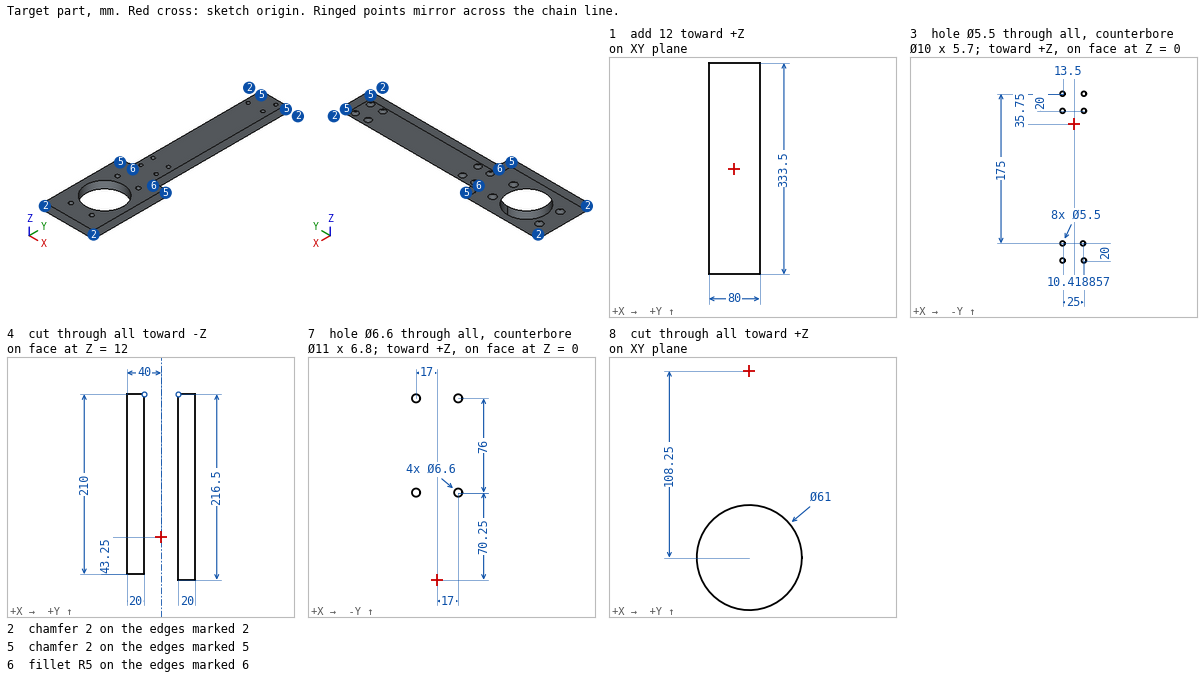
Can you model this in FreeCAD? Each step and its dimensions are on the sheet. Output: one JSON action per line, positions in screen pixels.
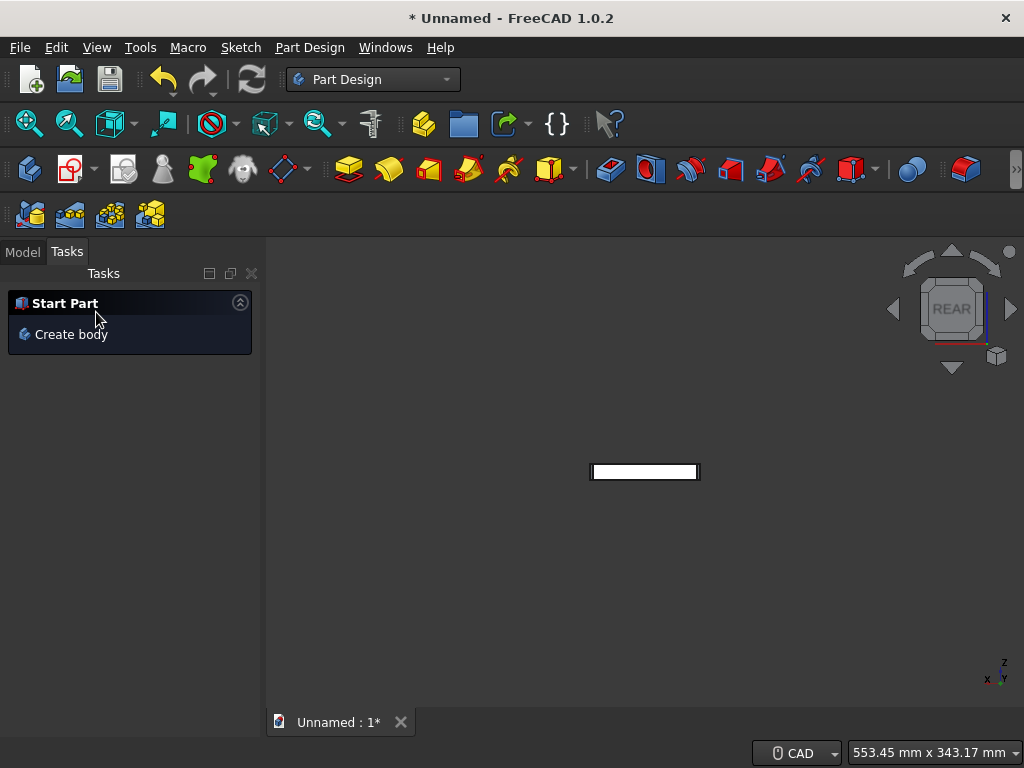
{"action": "key", "text": "5"}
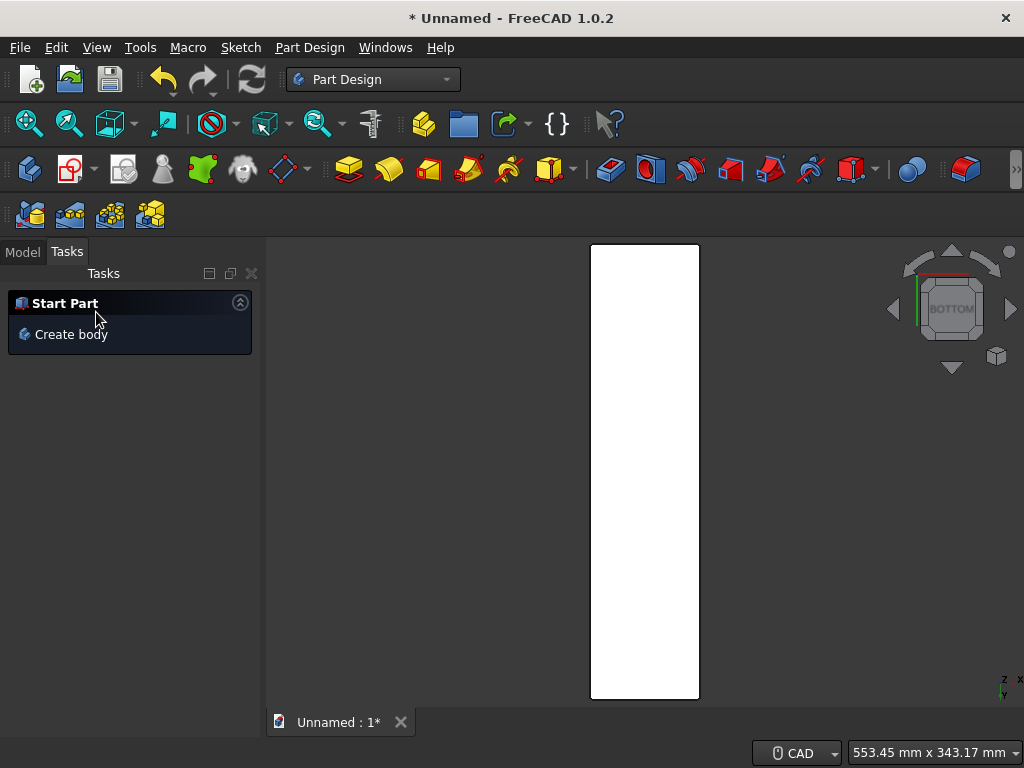
{"action": "left_click", "coordinate": [645, 602]}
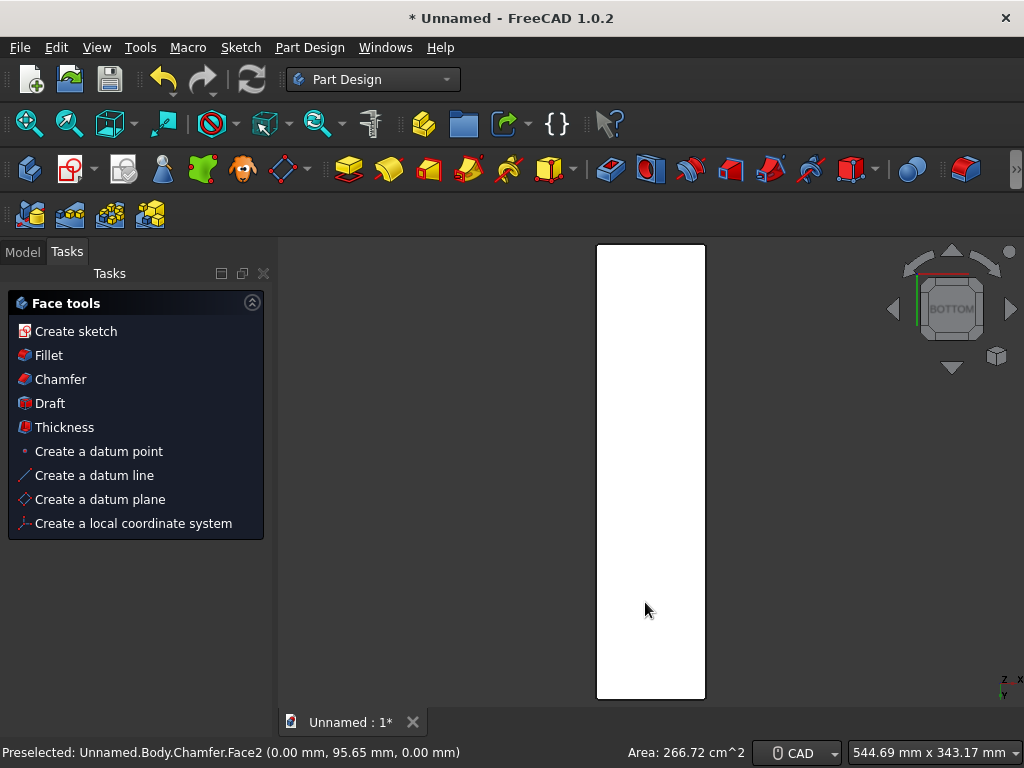
{"action": "left_click", "coordinate": [70, 170]}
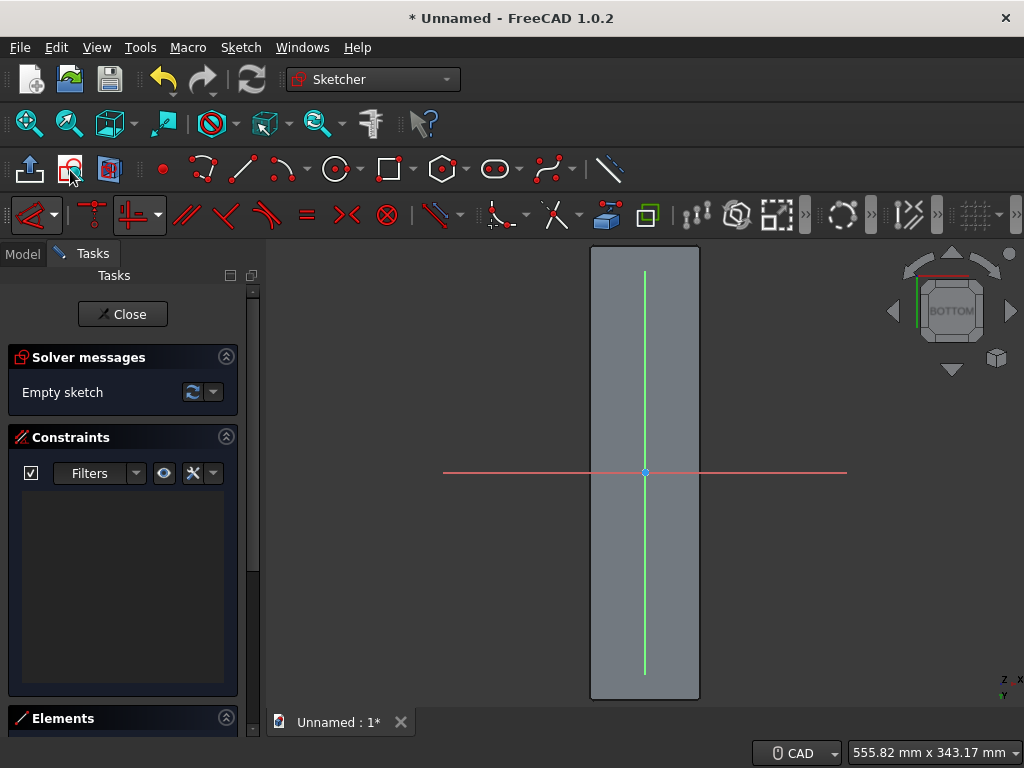
{"action": "scroll", "coordinate": [294, 267], "scroll_direction": "down", "scroll_amount": 1}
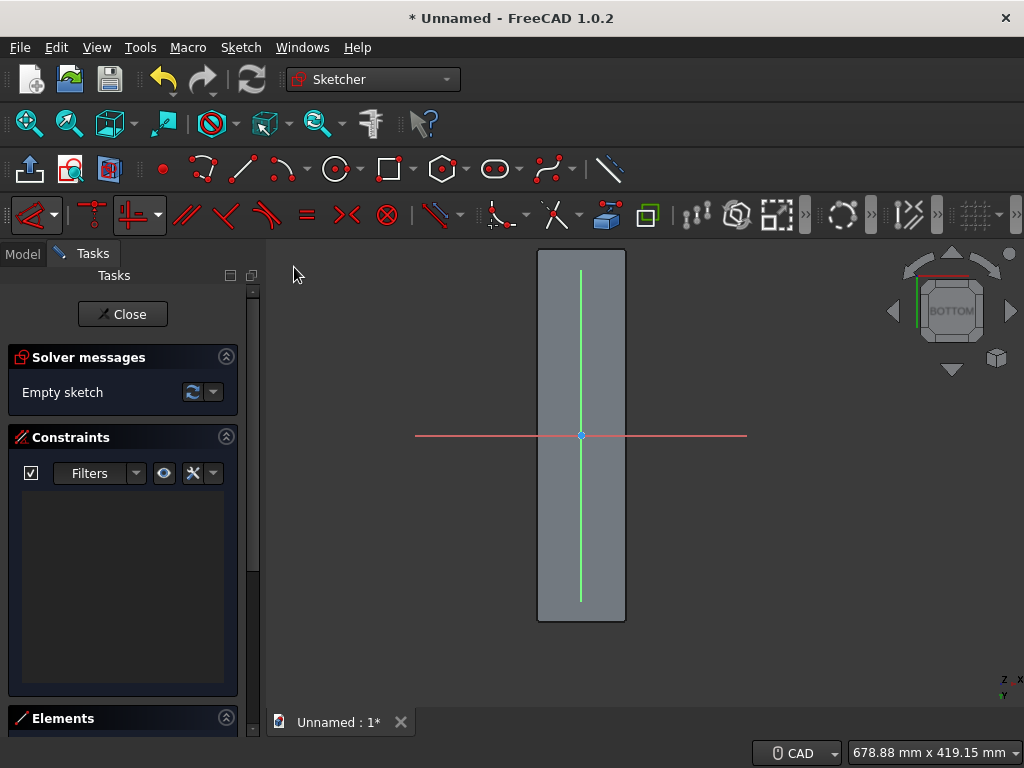
{"action": "key", "text": "g c"}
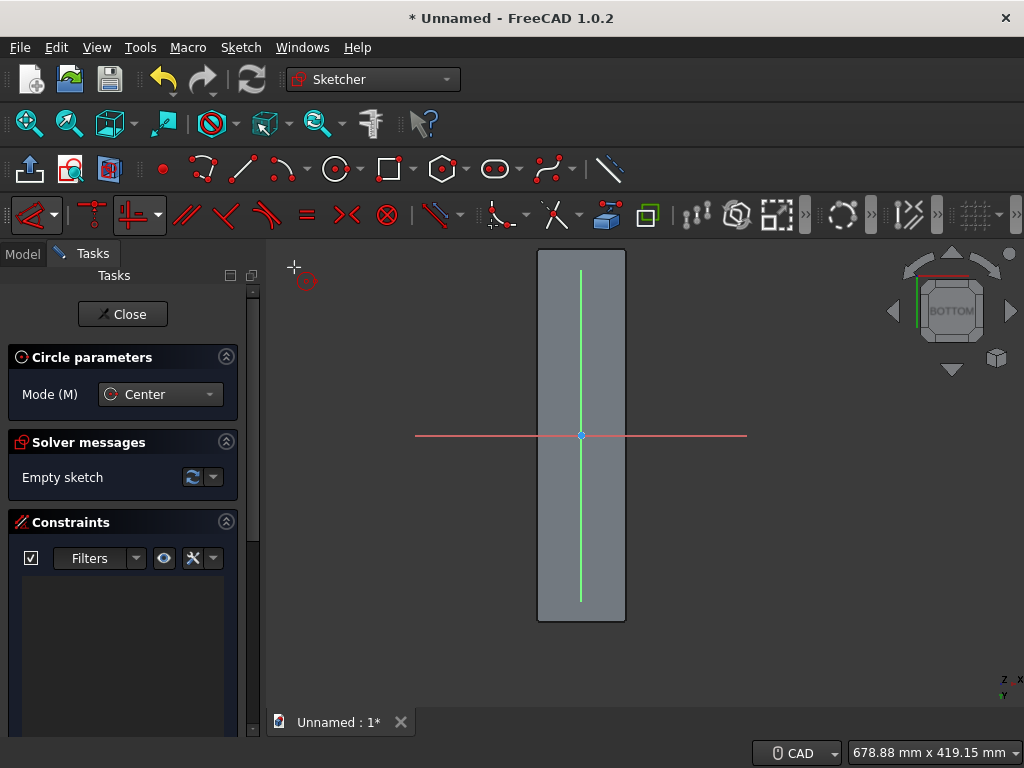
{"action": "scroll", "coordinate": [566, 396], "scroll_direction": "up", "scroll_amount": 10}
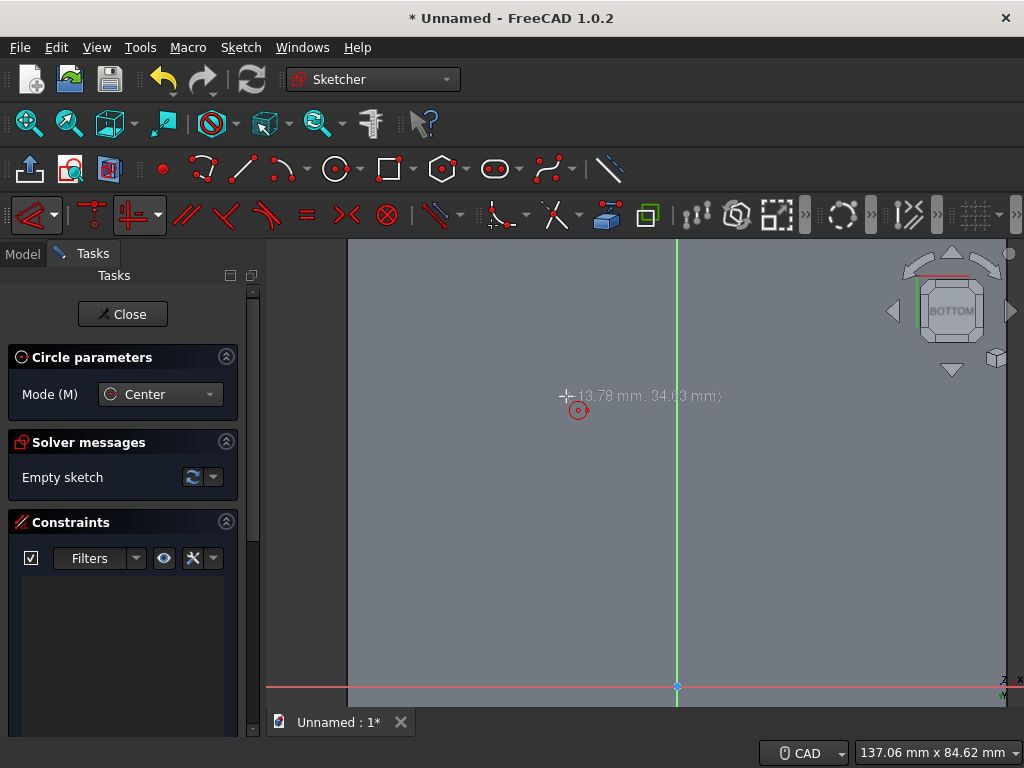
{"action": "scroll", "coordinate": [558, 330], "scroll_direction": "down", "scroll_amount": 9}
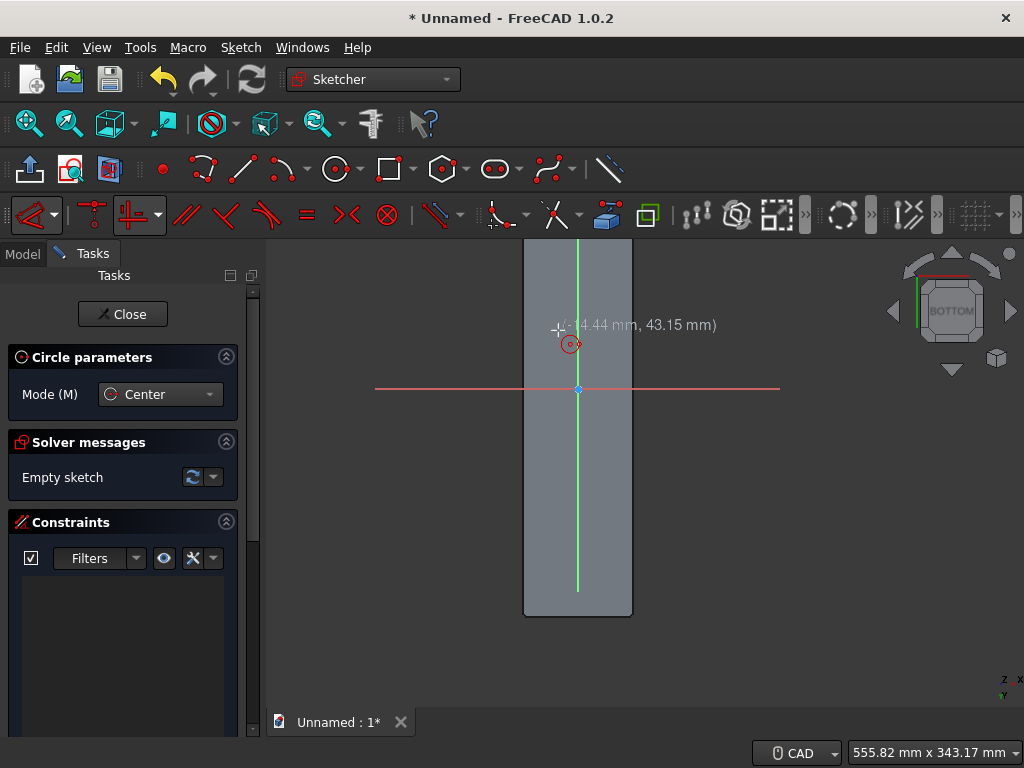
{"action": "left_click", "coordinate": [560, 340]}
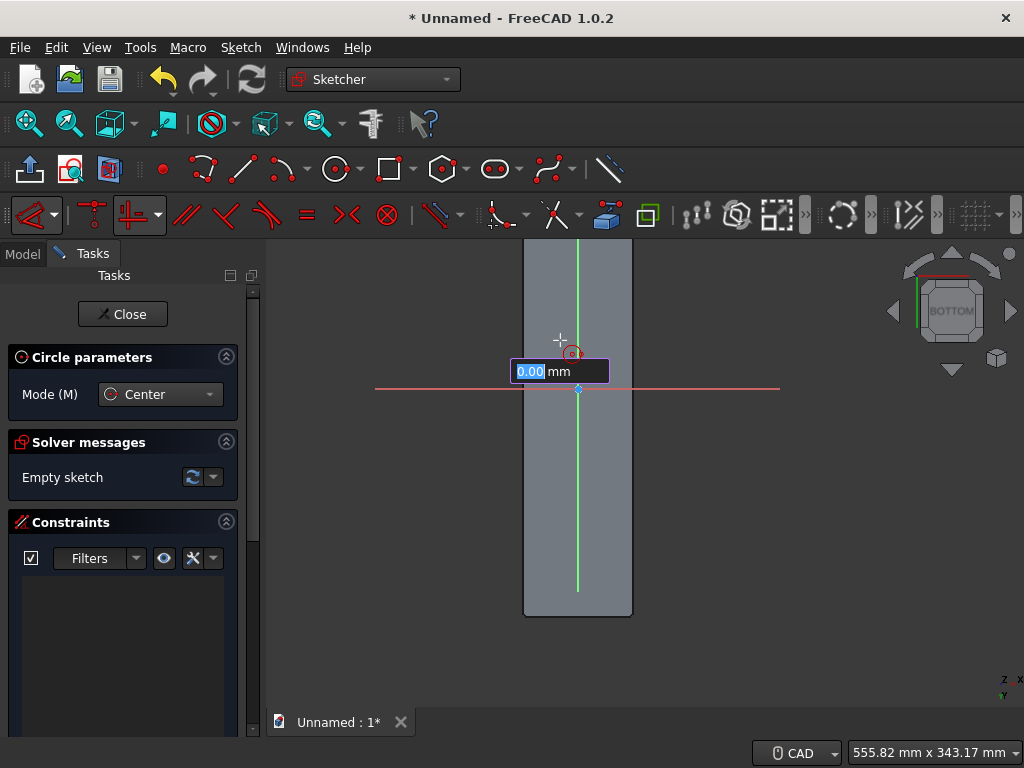
{"action": "scroll", "coordinate": [562, 338], "scroll_direction": "up", "scroll_amount": 8}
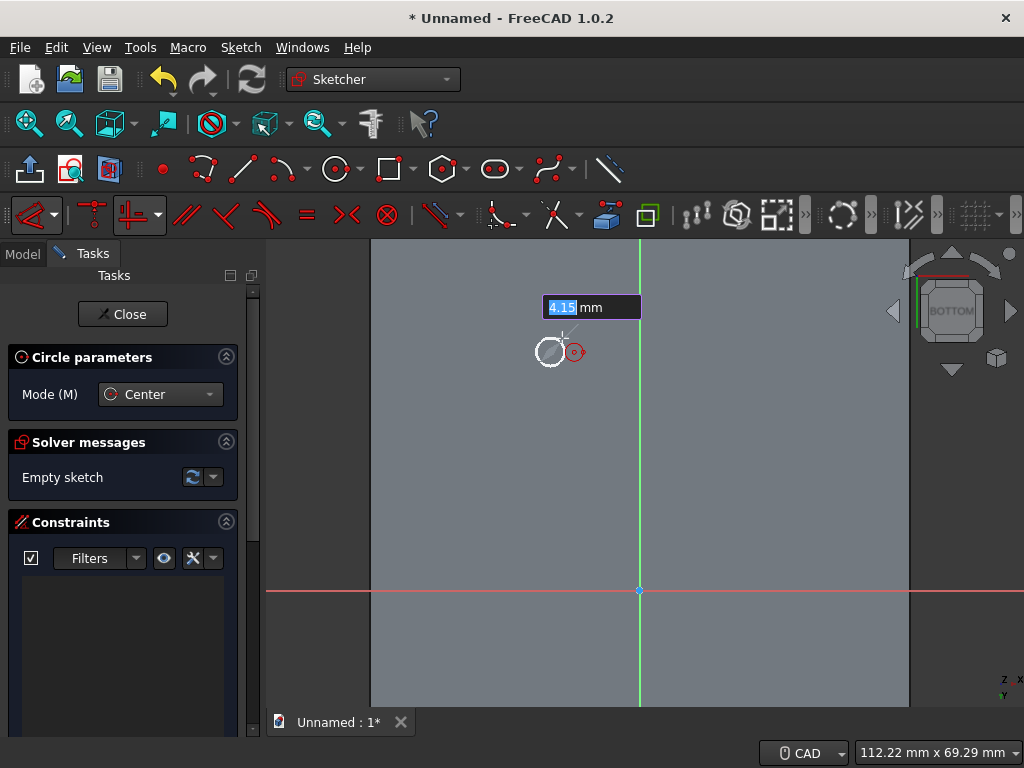
{"action": "left_click", "coordinate": [562, 336]}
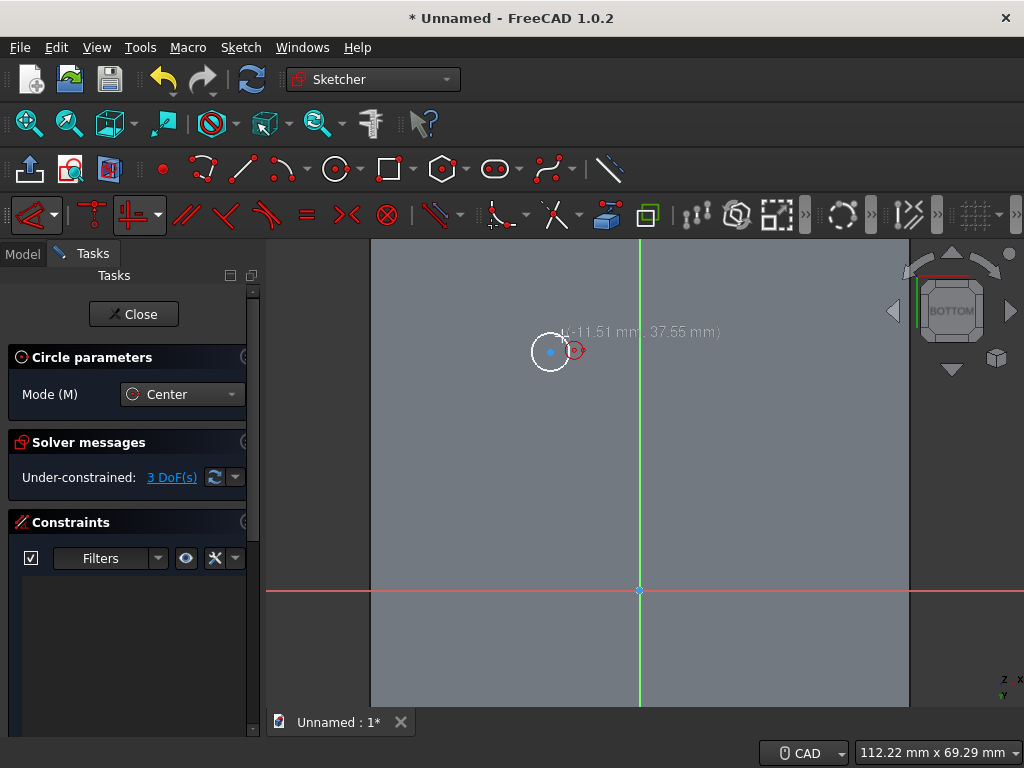
{"action": "scroll", "coordinate": [562, 338], "scroll_direction": "down", "scroll_amount": 8}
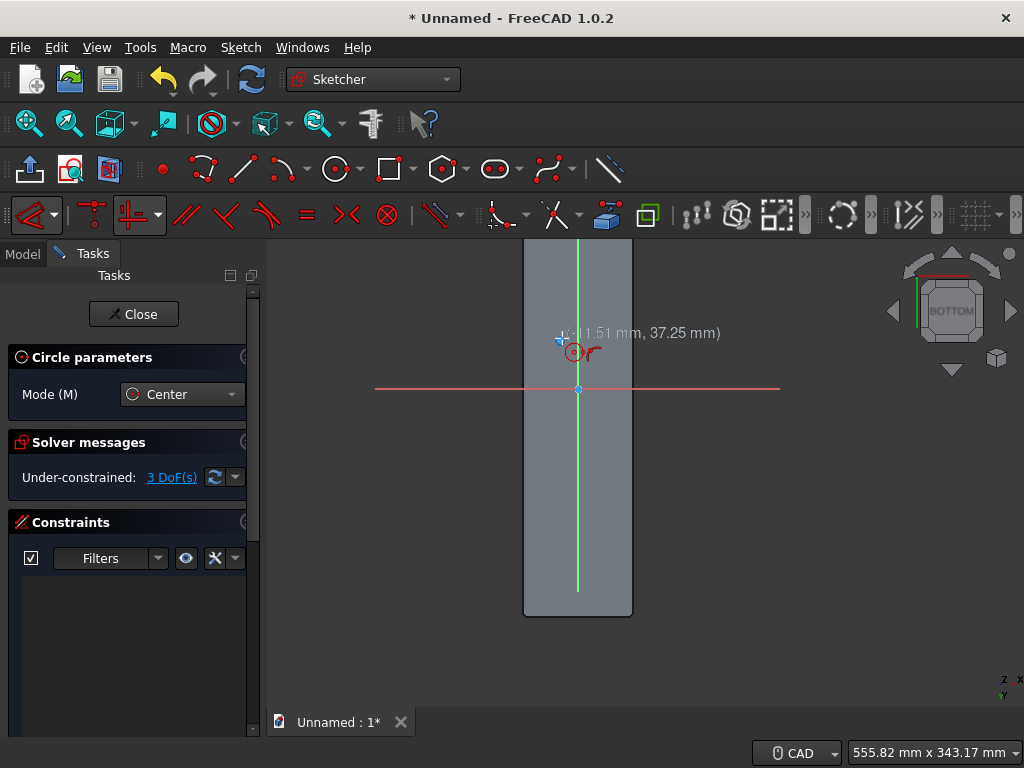
{"action": "scroll", "coordinate": [560, 579], "scroll_direction": "up", "scroll_amount": 9}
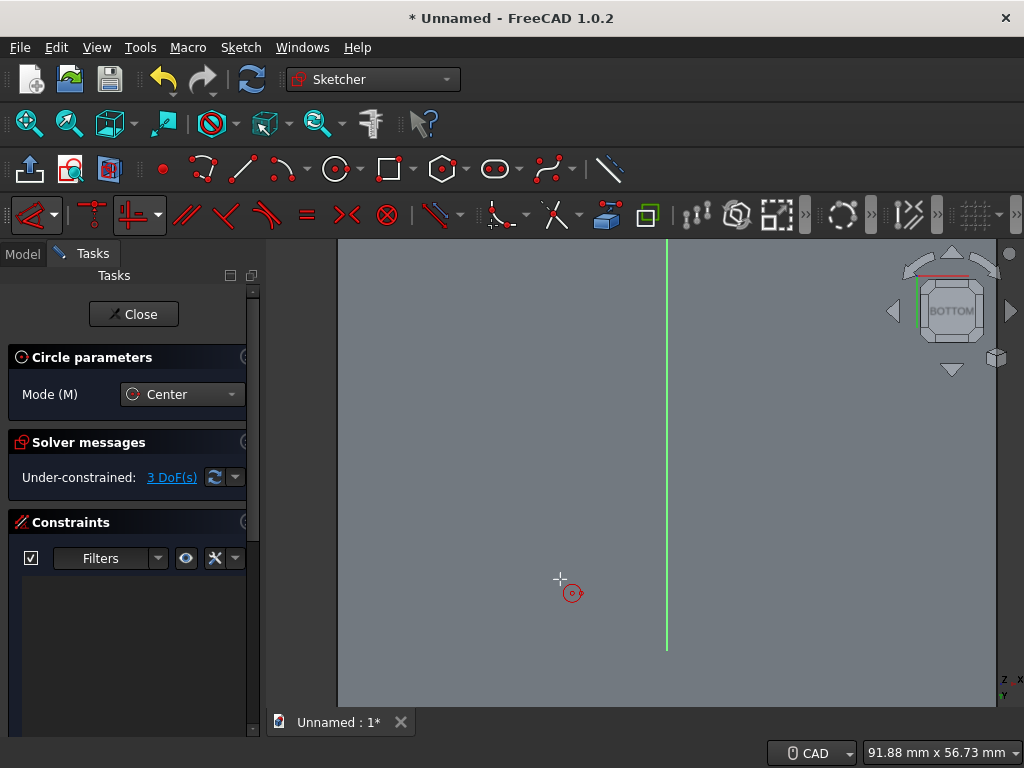
{"action": "scroll", "coordinate": [560, 579], "scroll_direction": "down", "scroll_amount": 9}